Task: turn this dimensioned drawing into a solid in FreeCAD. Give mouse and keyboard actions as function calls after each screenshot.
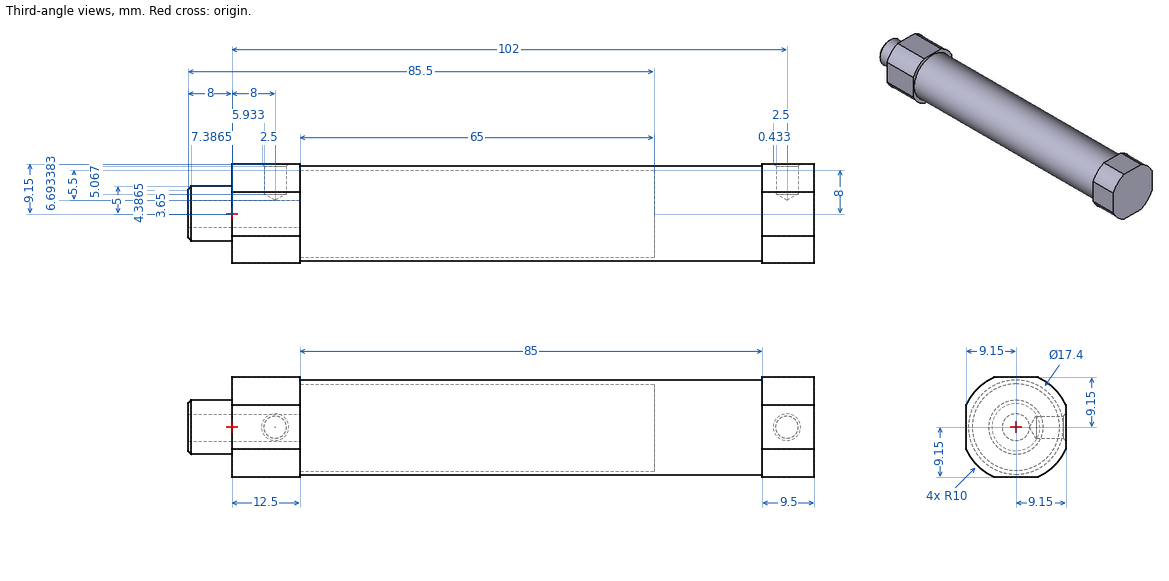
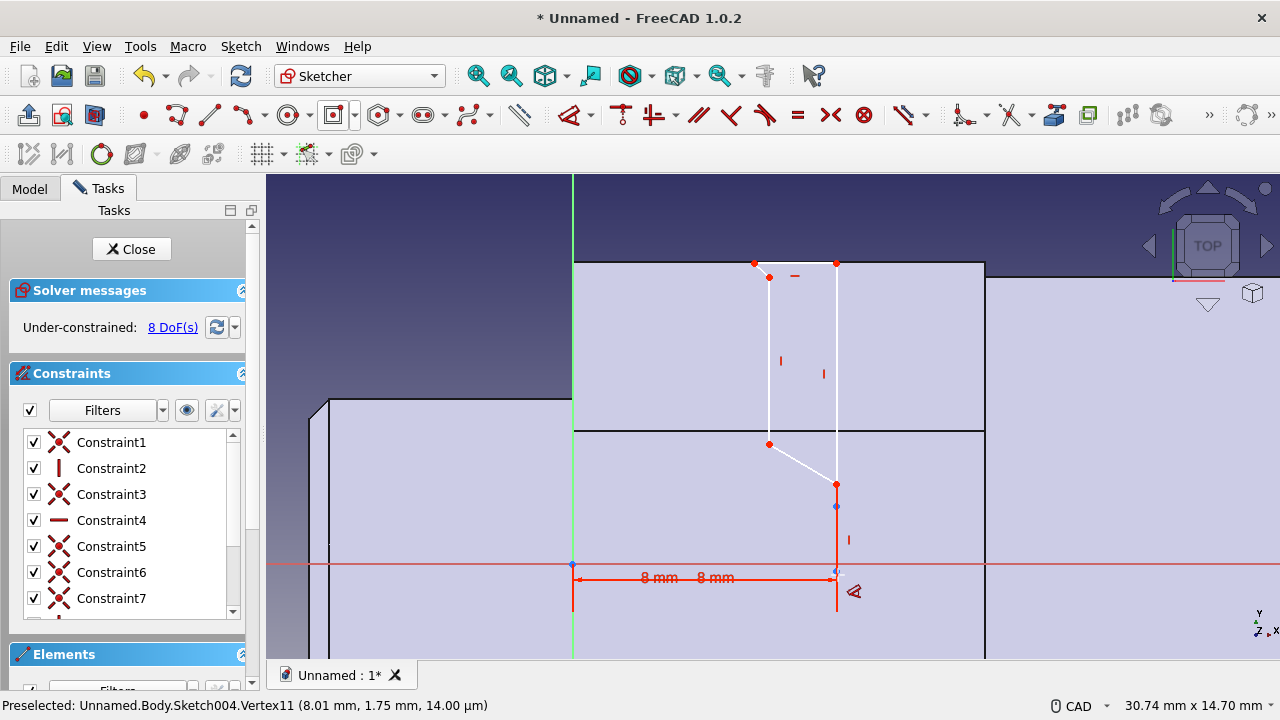
click(812, 263)
click(796, 229)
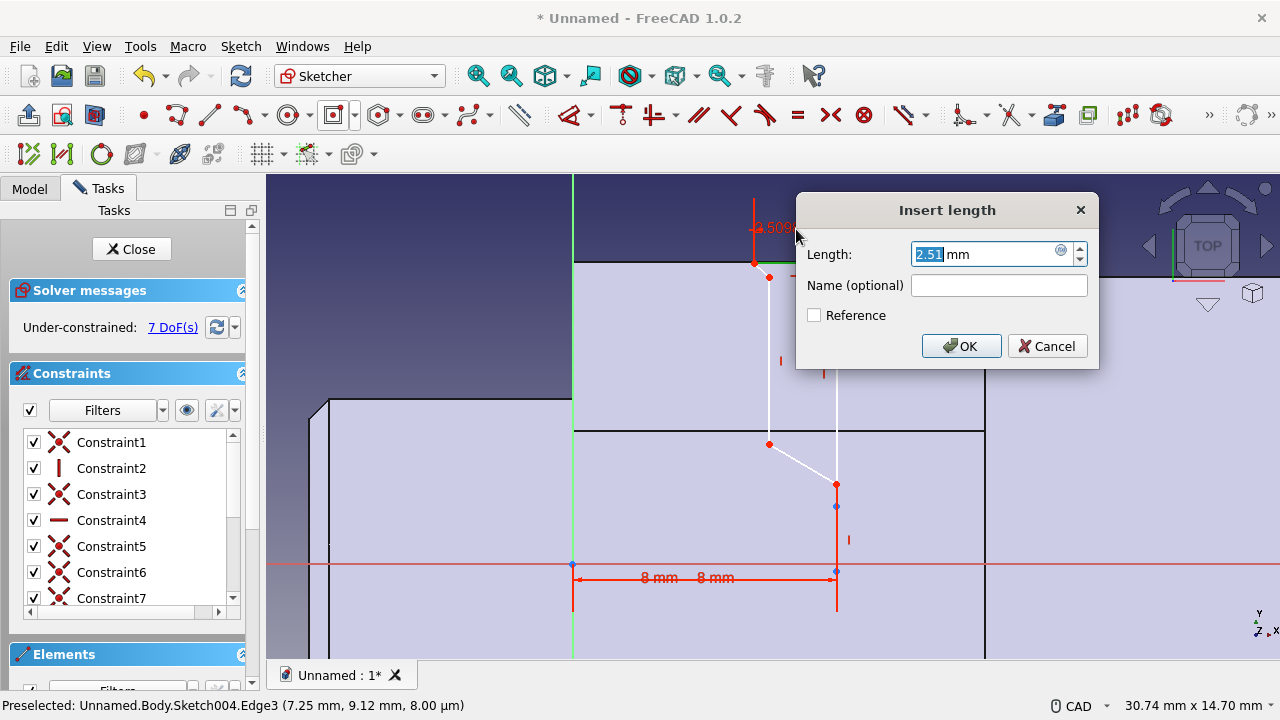
text(2.5)
key(Return)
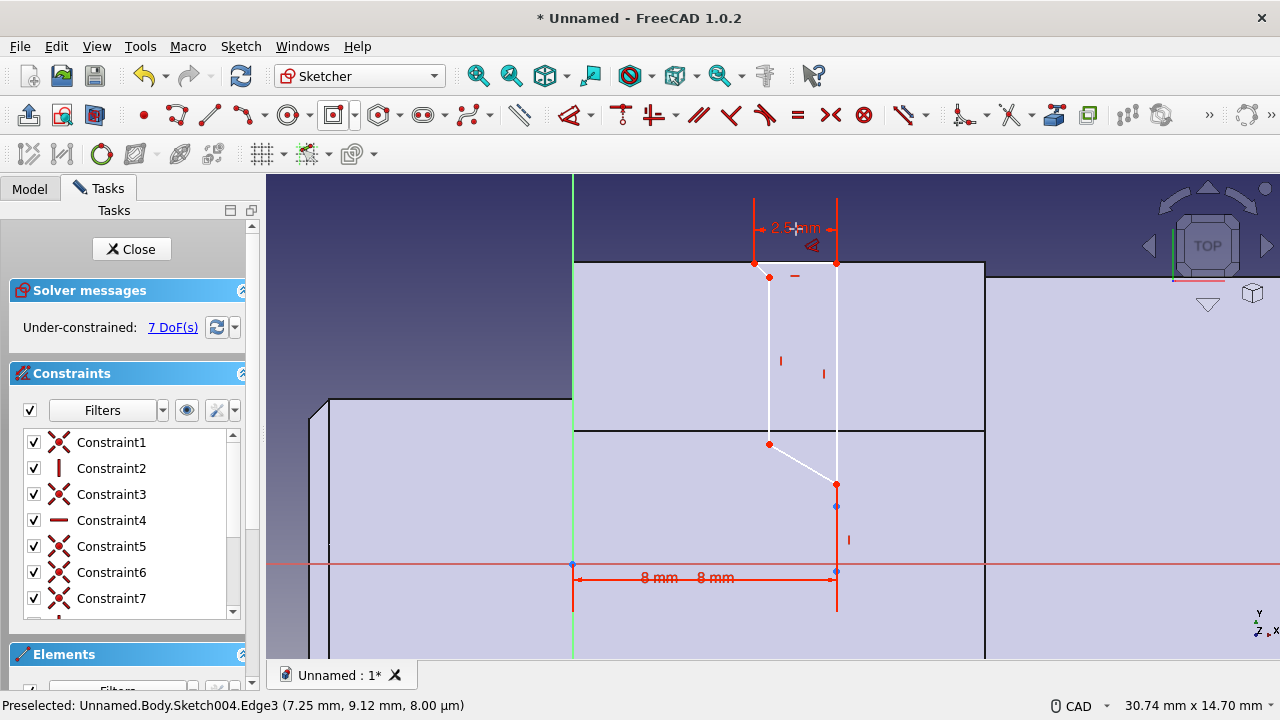
click(769, 328)
click(803, 361)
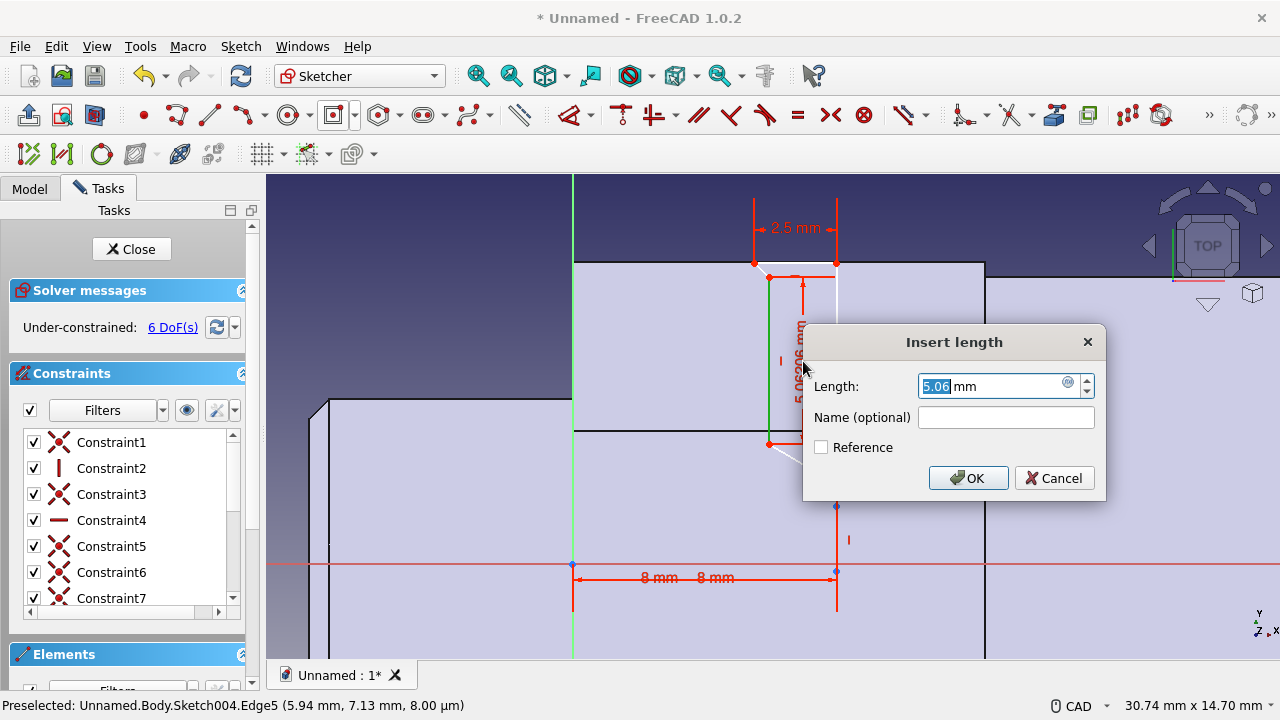
text(5.067)
key(Return)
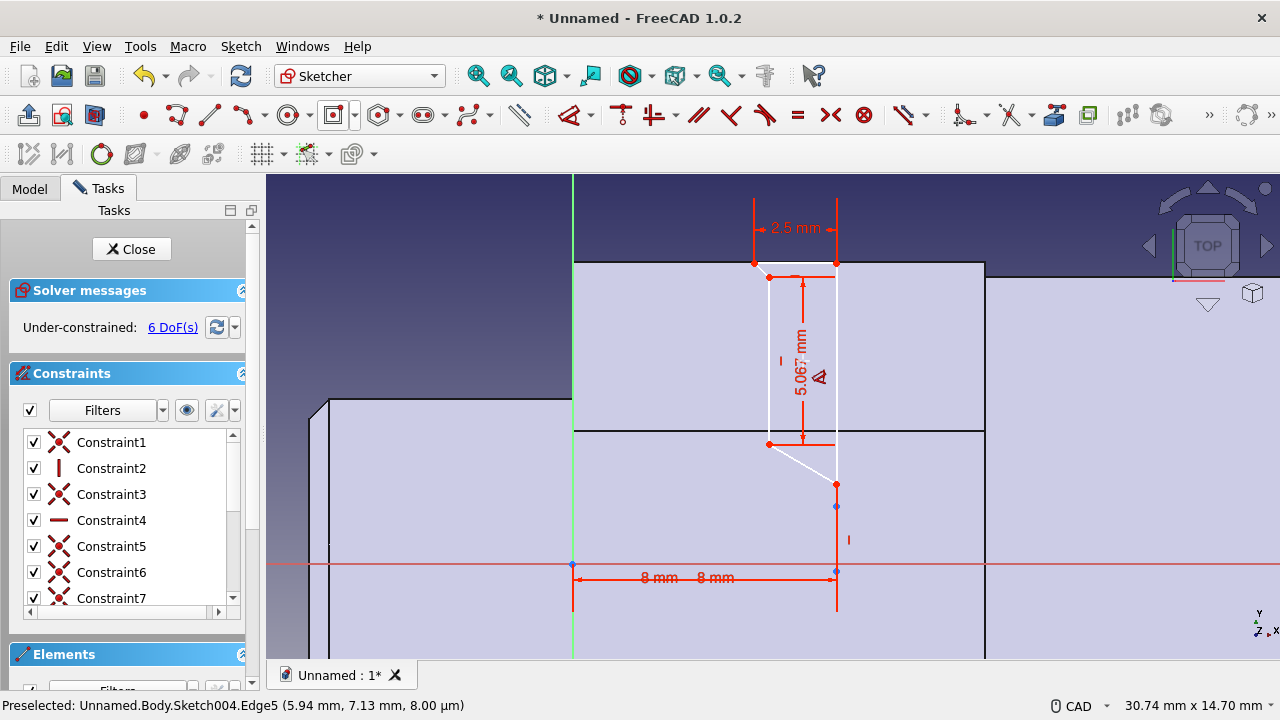
click(769, 445)
click(539, 504)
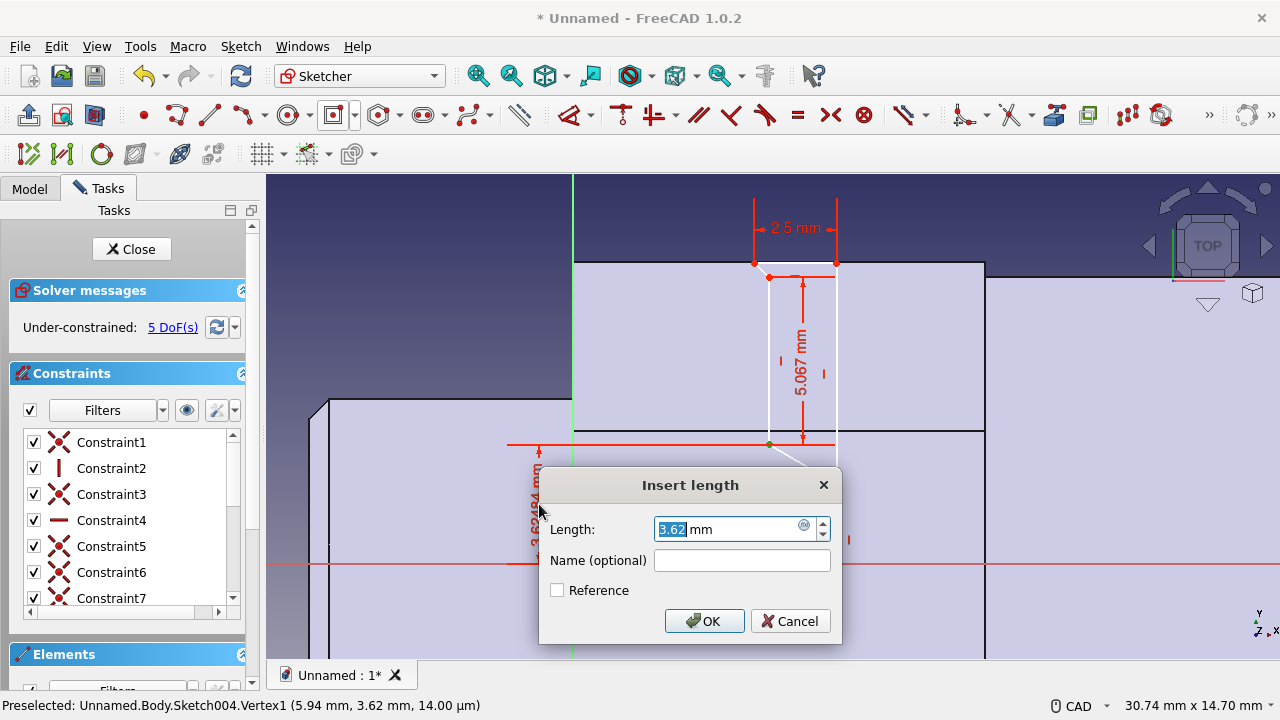
text(3.65)
key(Return)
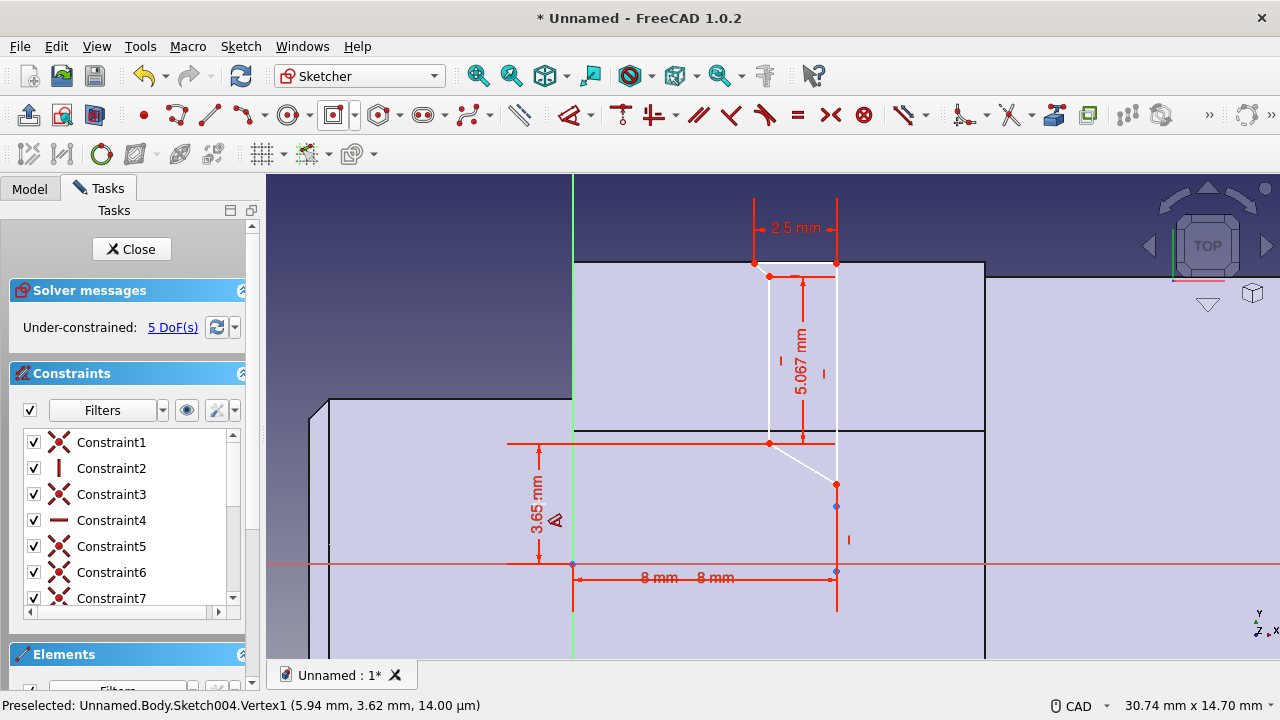
click(837, 263)
click(871, 414)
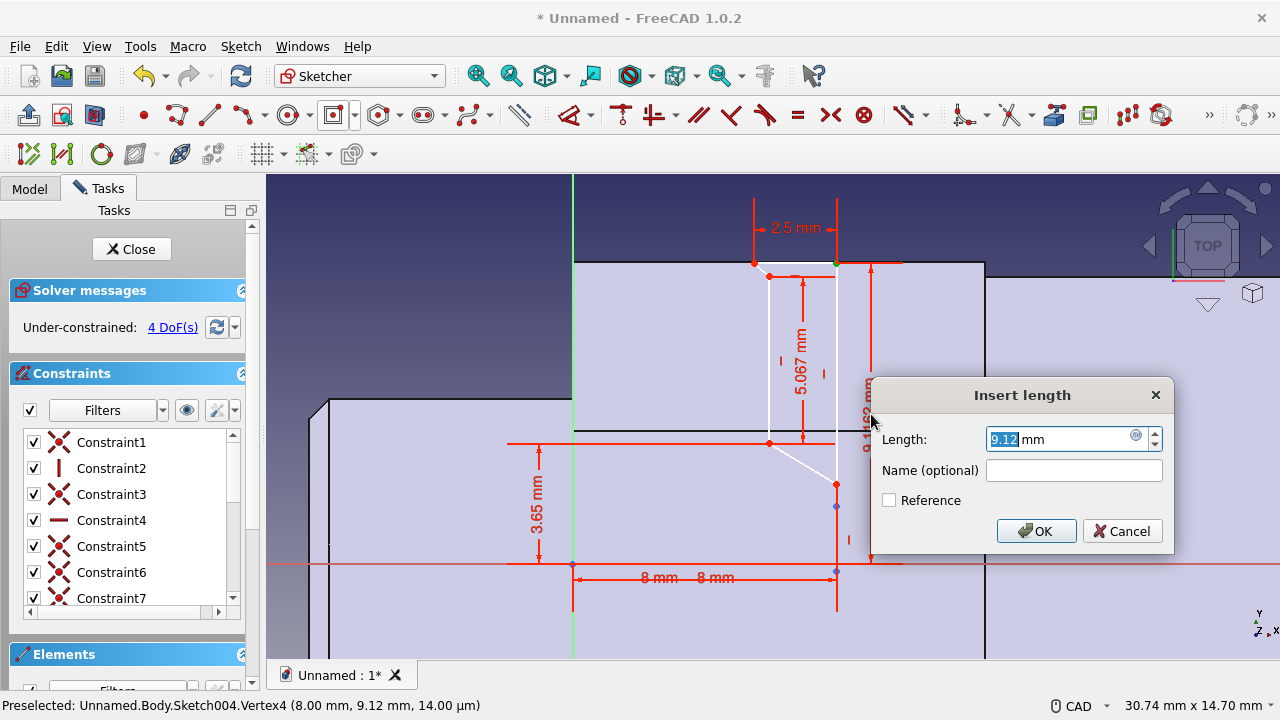
text(9.15)
key(Return)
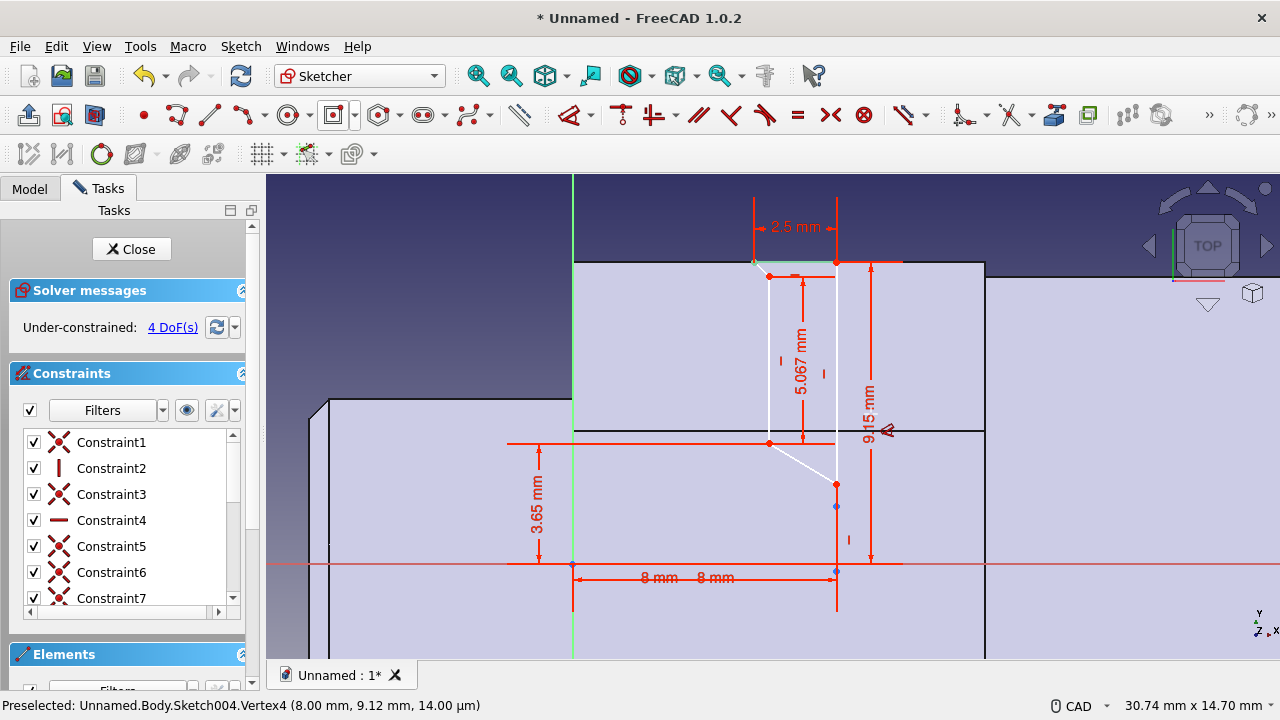
click(769, 444)
click(671, 410)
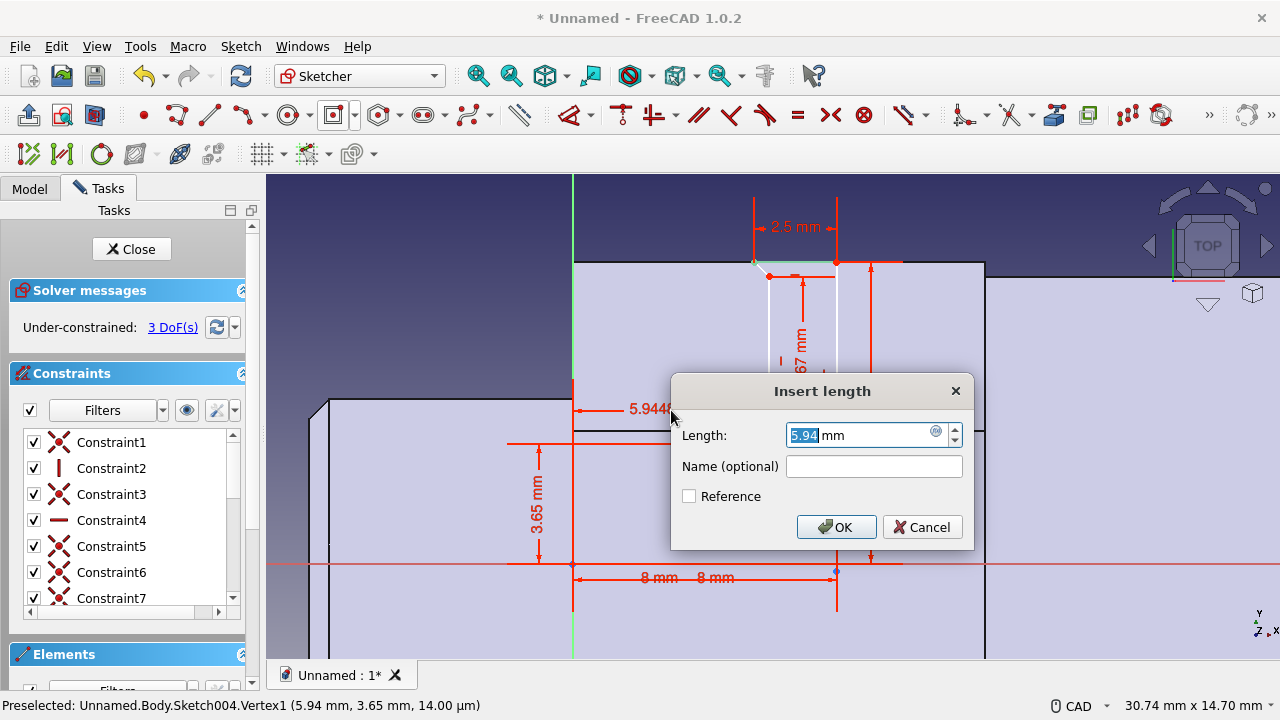
text(5.933)
key(Return)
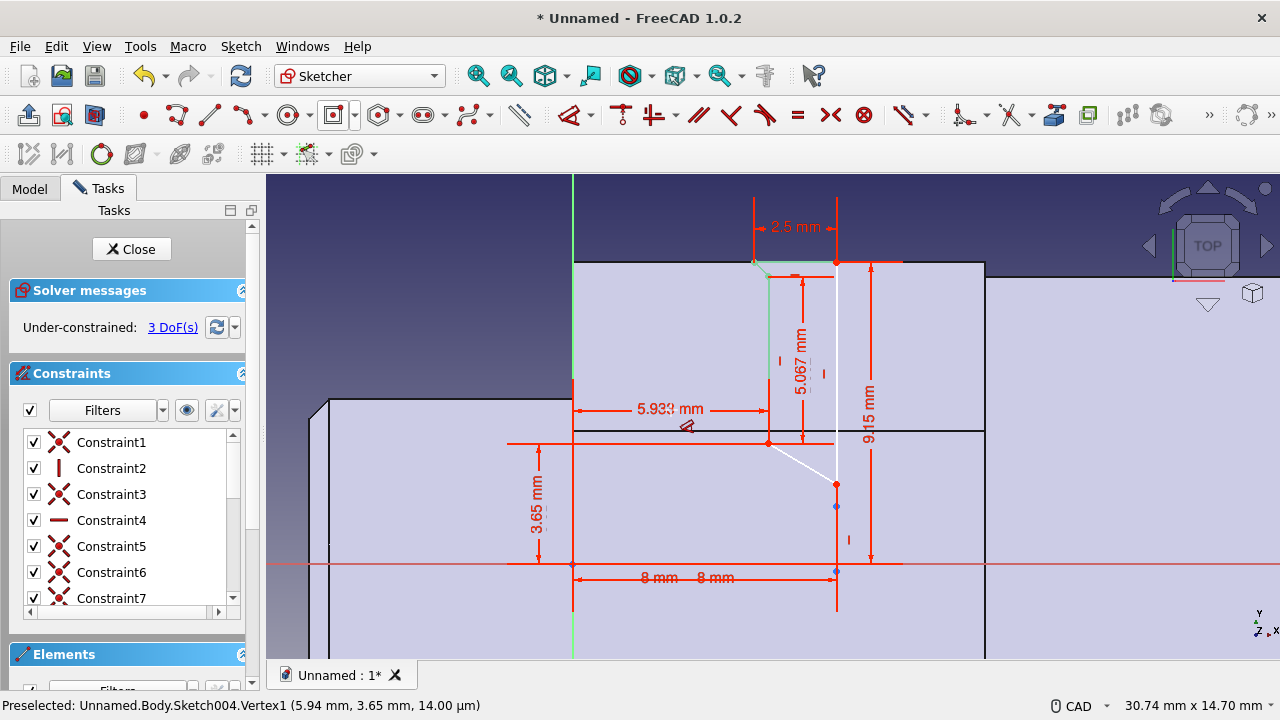
click(837, 418)
click(871, 322)